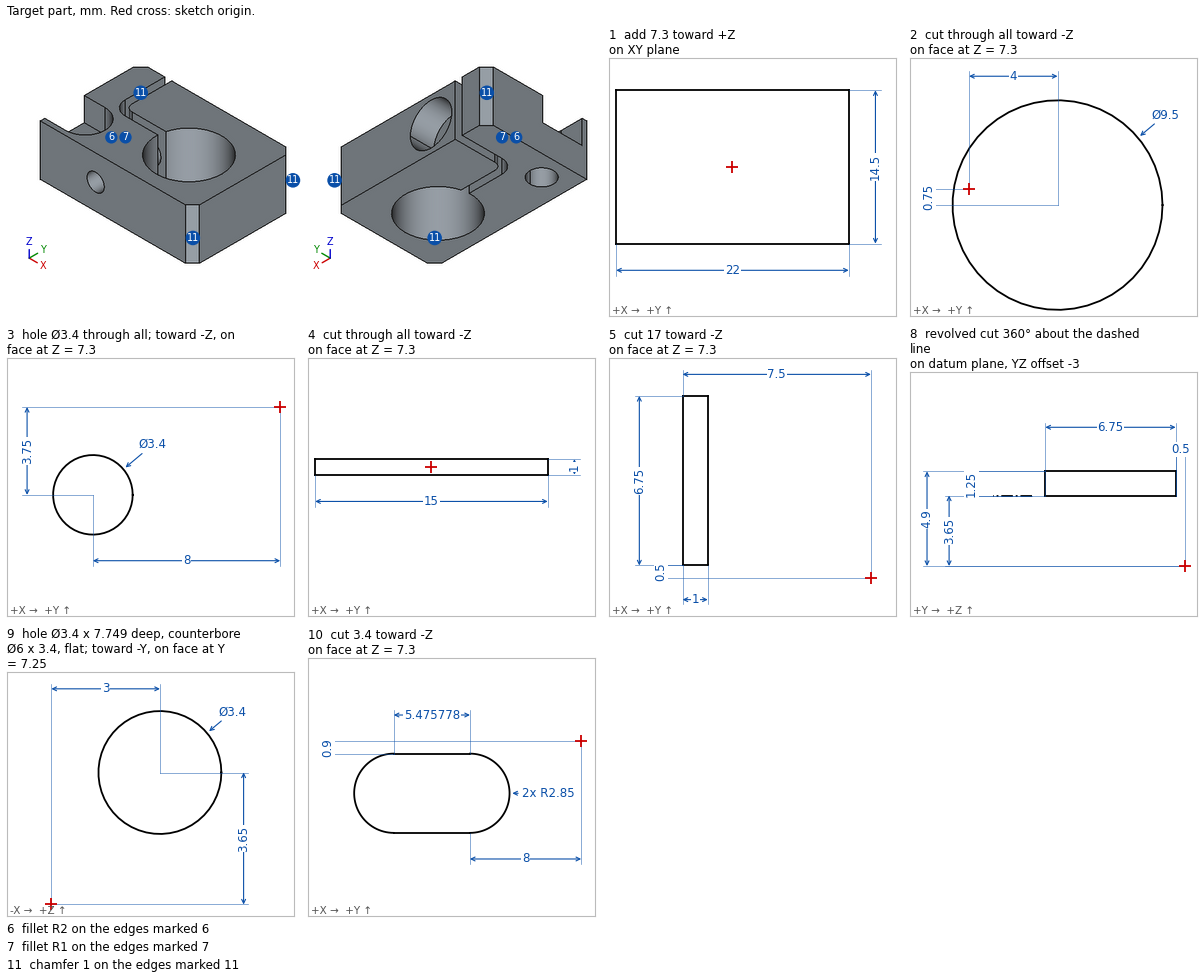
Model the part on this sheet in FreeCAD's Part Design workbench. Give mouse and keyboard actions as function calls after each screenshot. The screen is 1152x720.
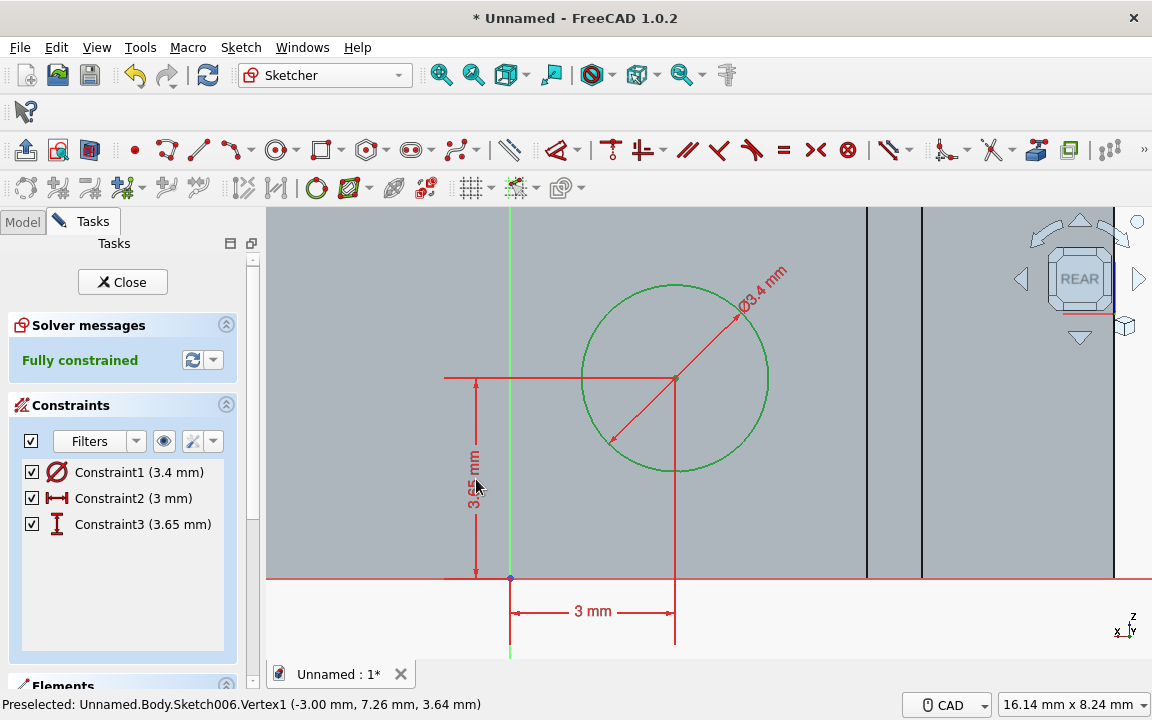
click(123, 282)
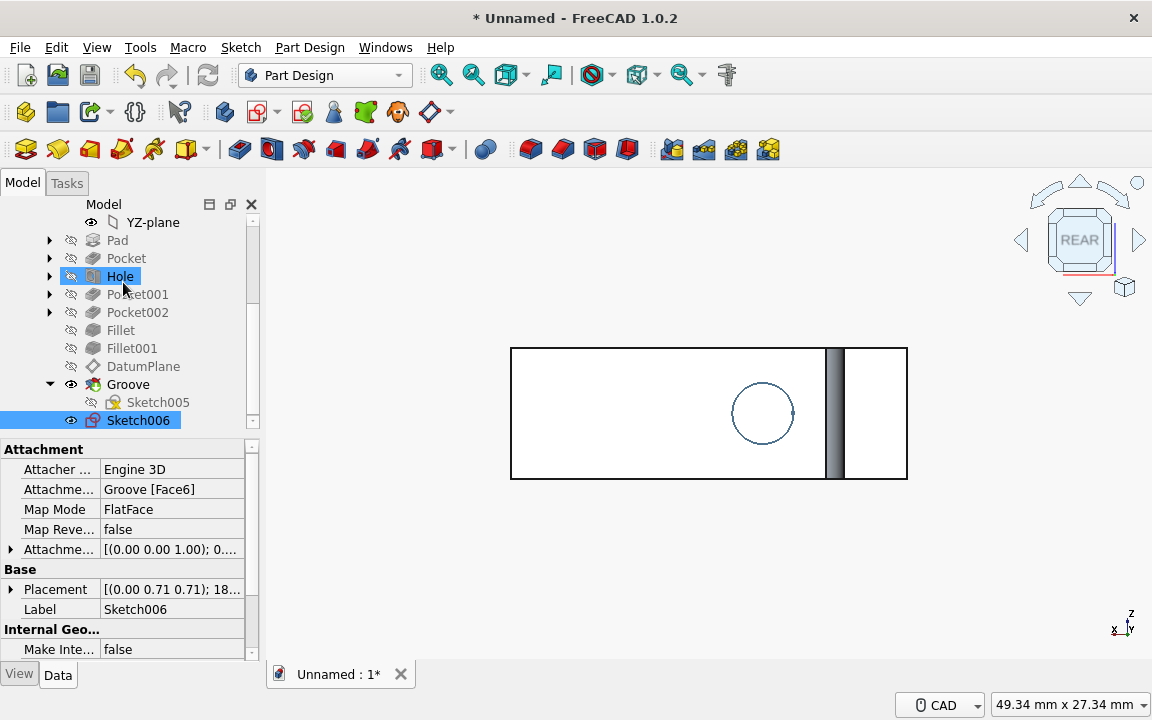
click(272, 150)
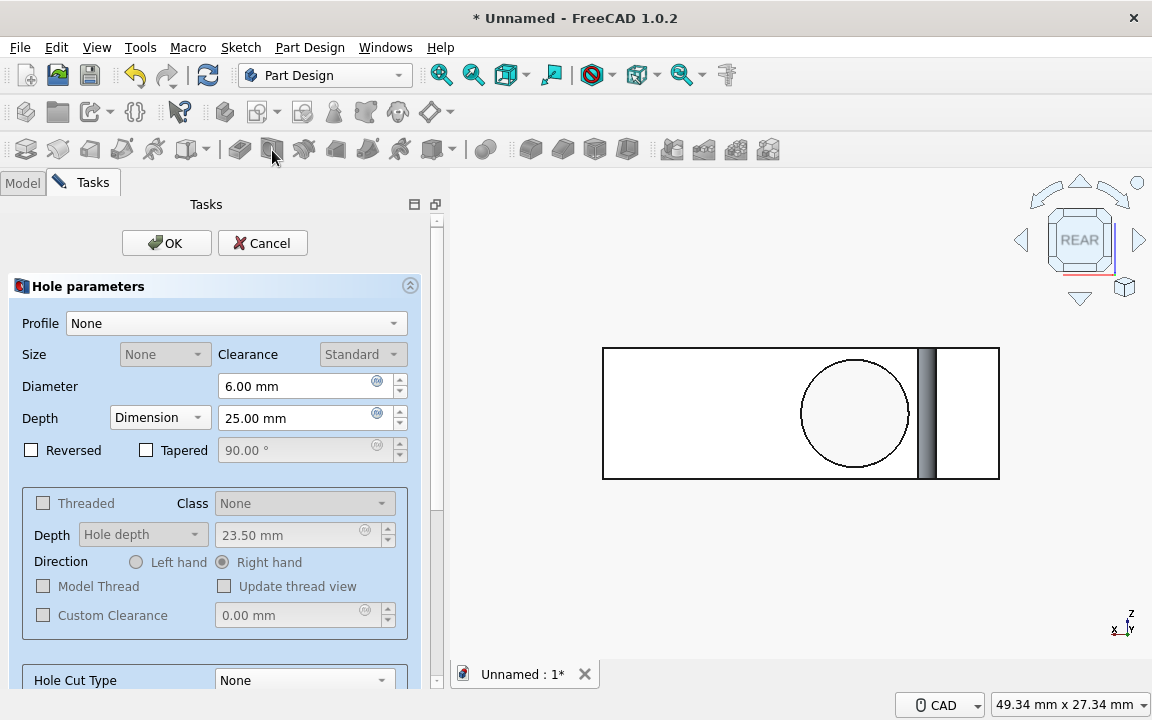
triple_click(305, 386)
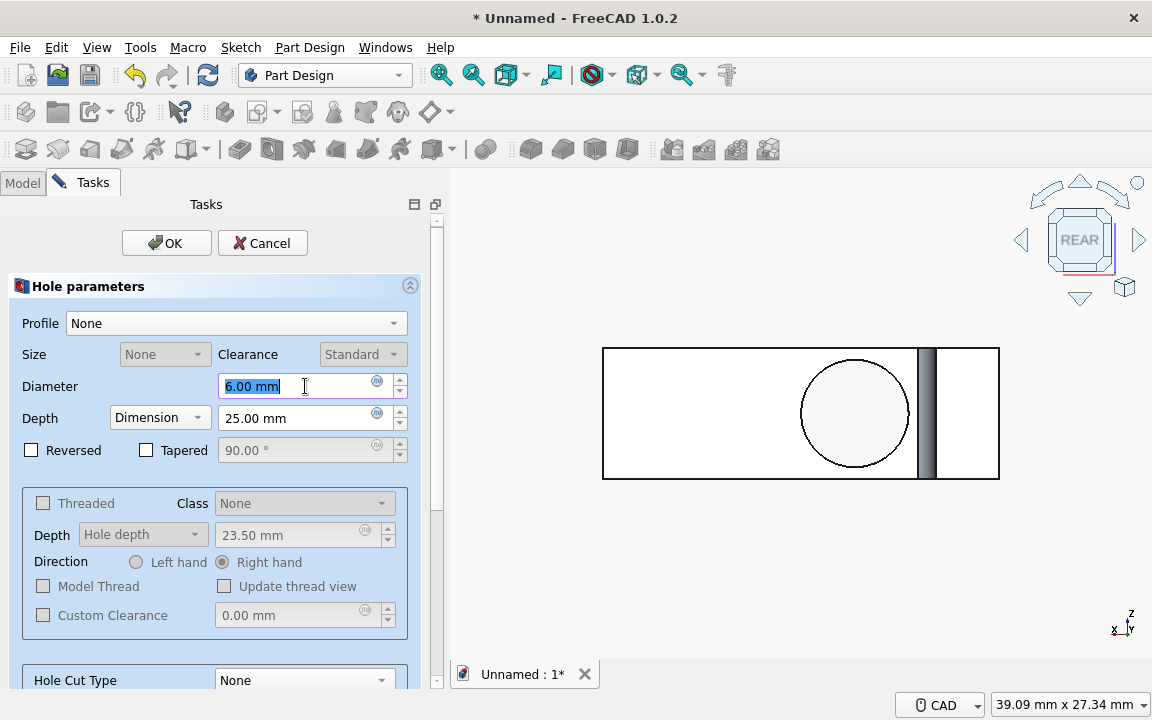
text(3.4)
key(Tab)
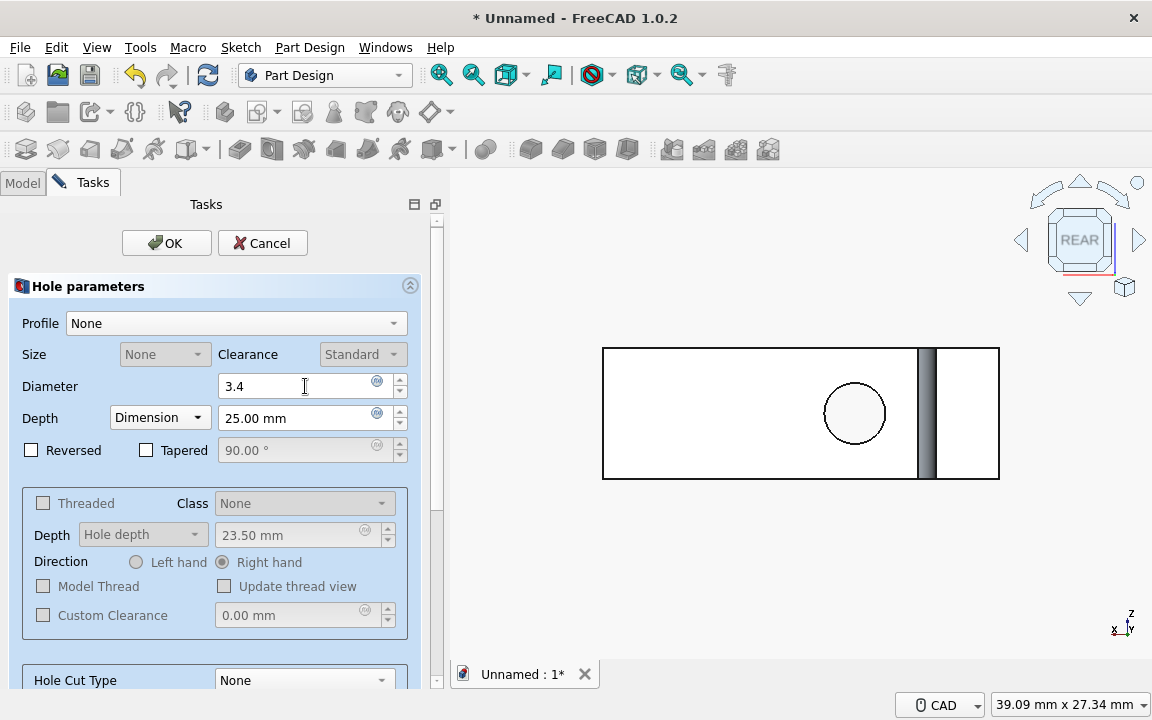
triple_click(305, 418)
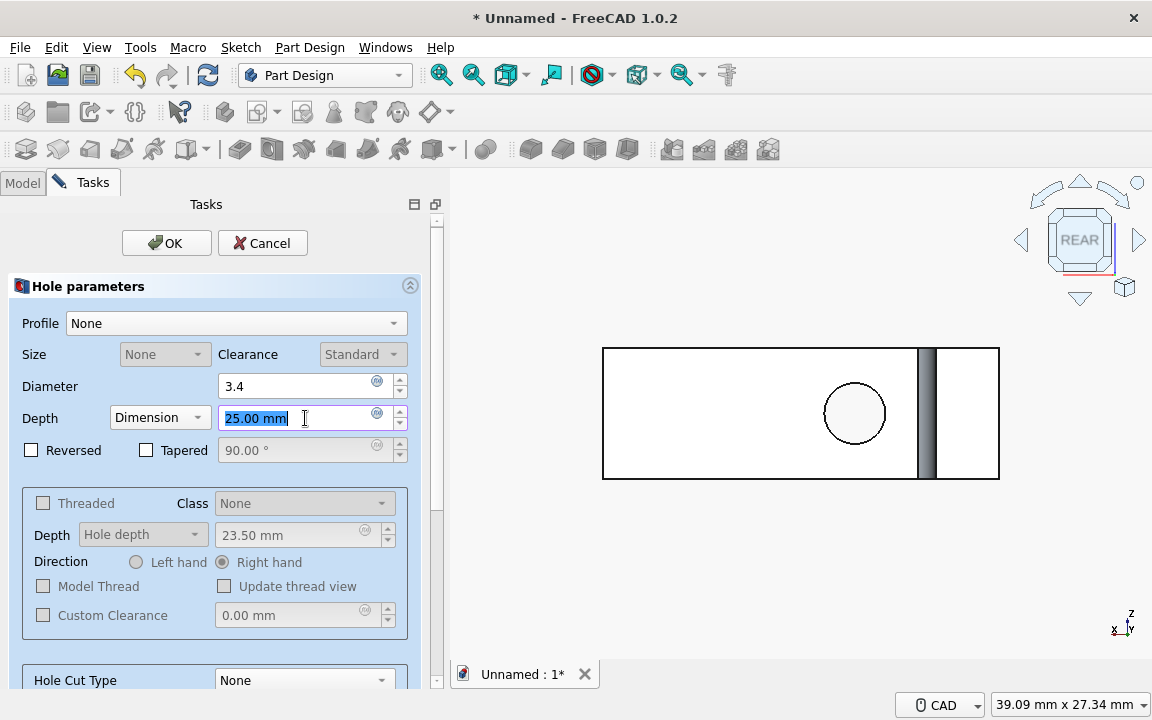
text(7.749)
key(Tab)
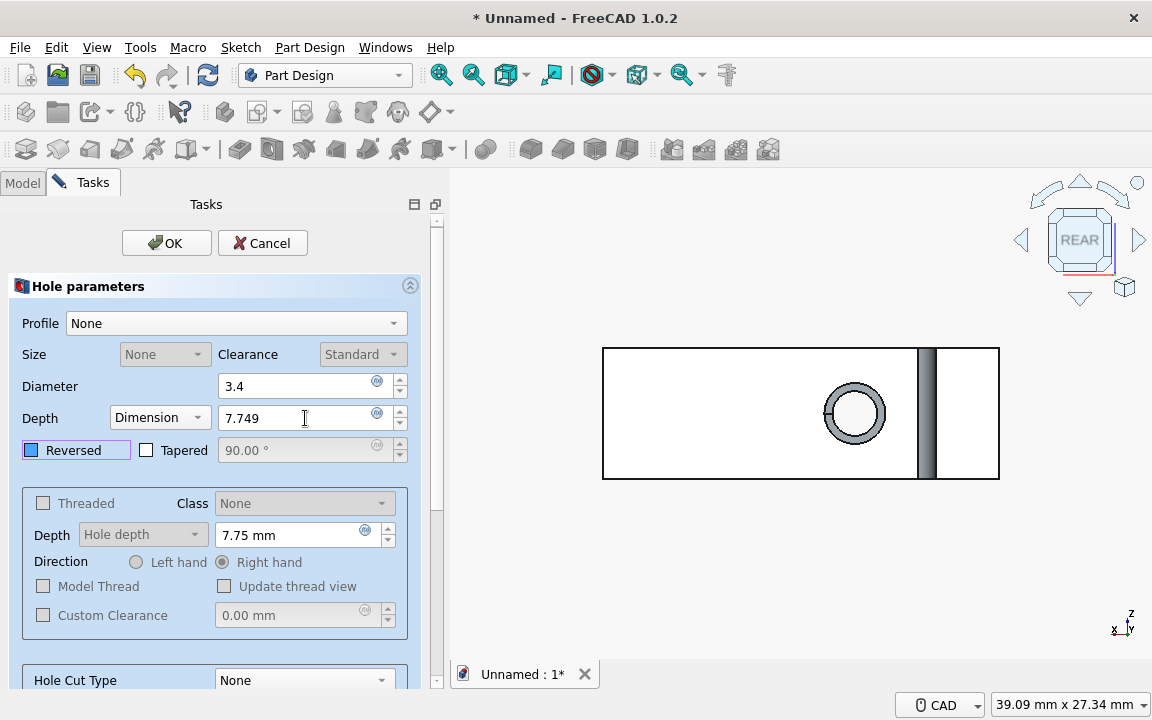
scroll(437, 451, down, 2)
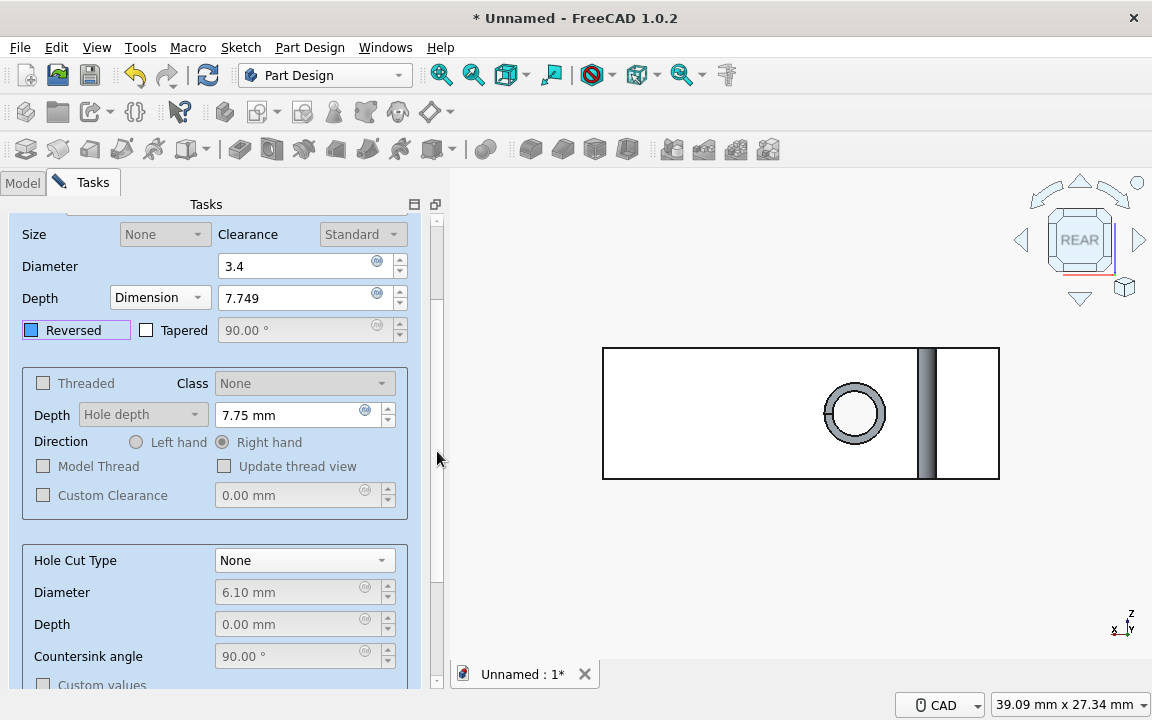
click(306, 560)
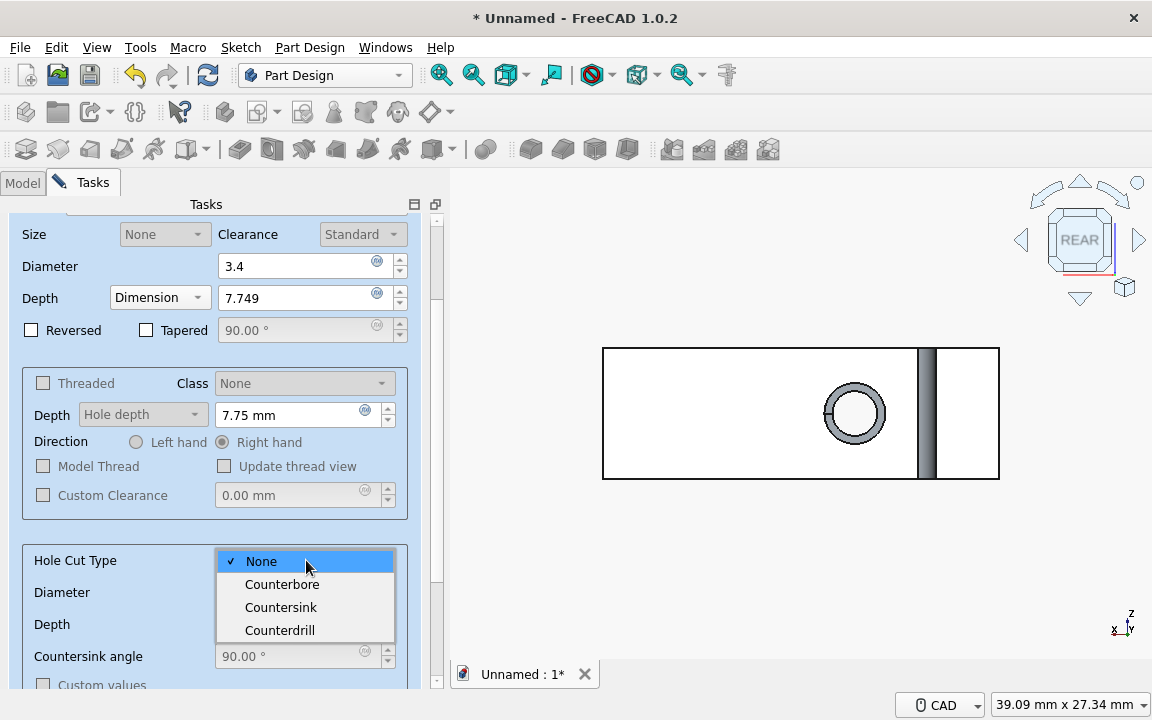
click(304, 584)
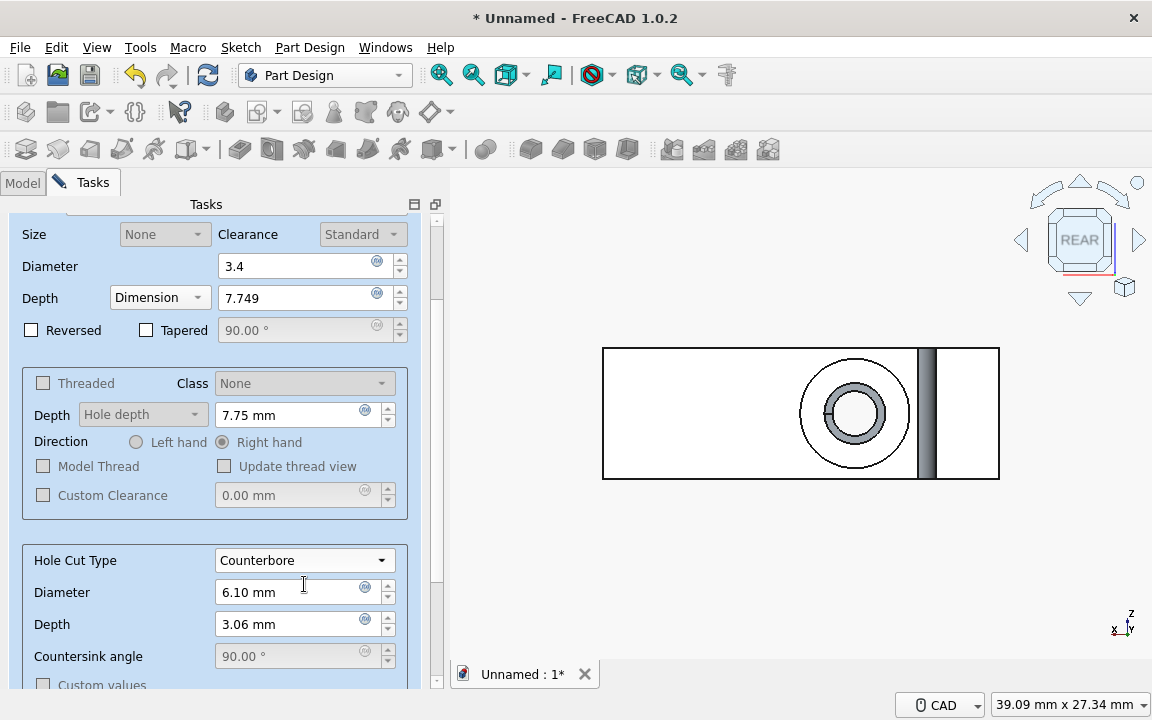
triple_click(298, 592)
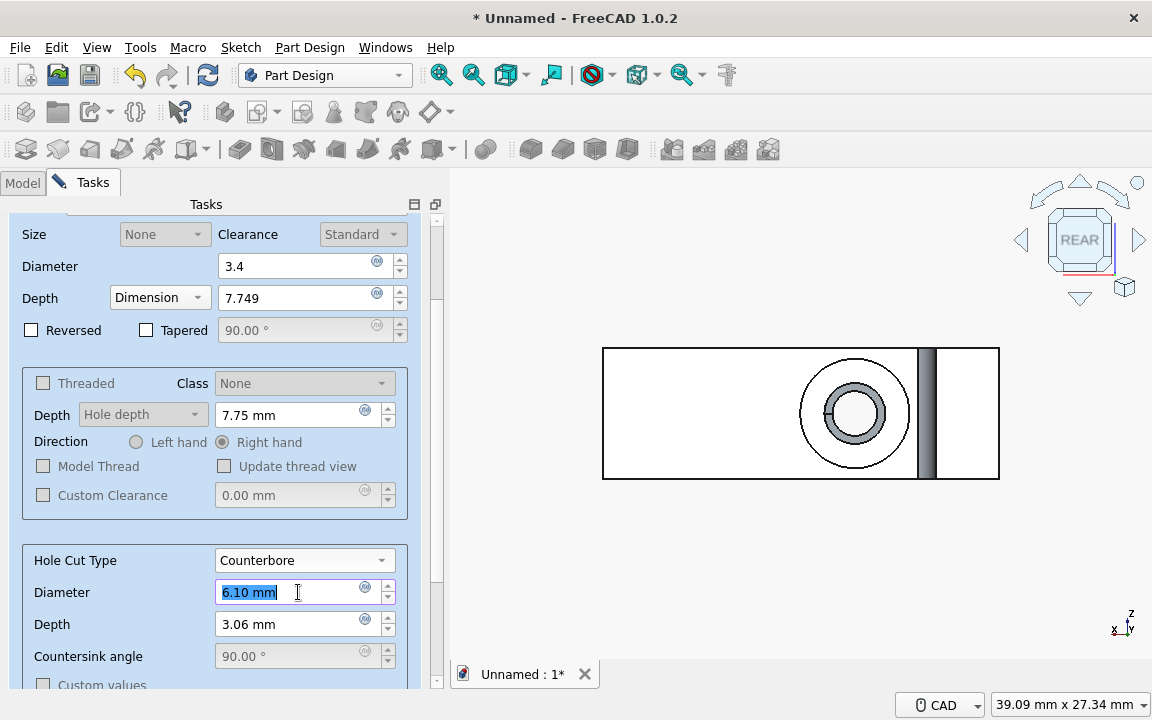
text(6)
key(Tab)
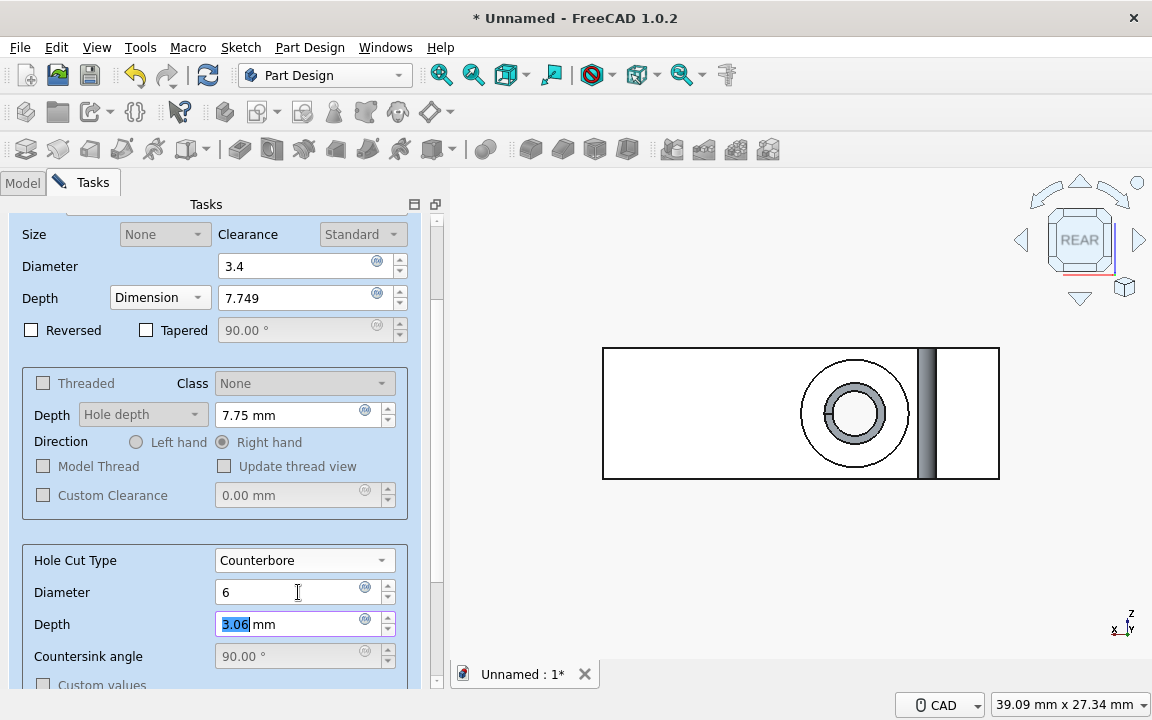
text(3.4)
key(Tab)